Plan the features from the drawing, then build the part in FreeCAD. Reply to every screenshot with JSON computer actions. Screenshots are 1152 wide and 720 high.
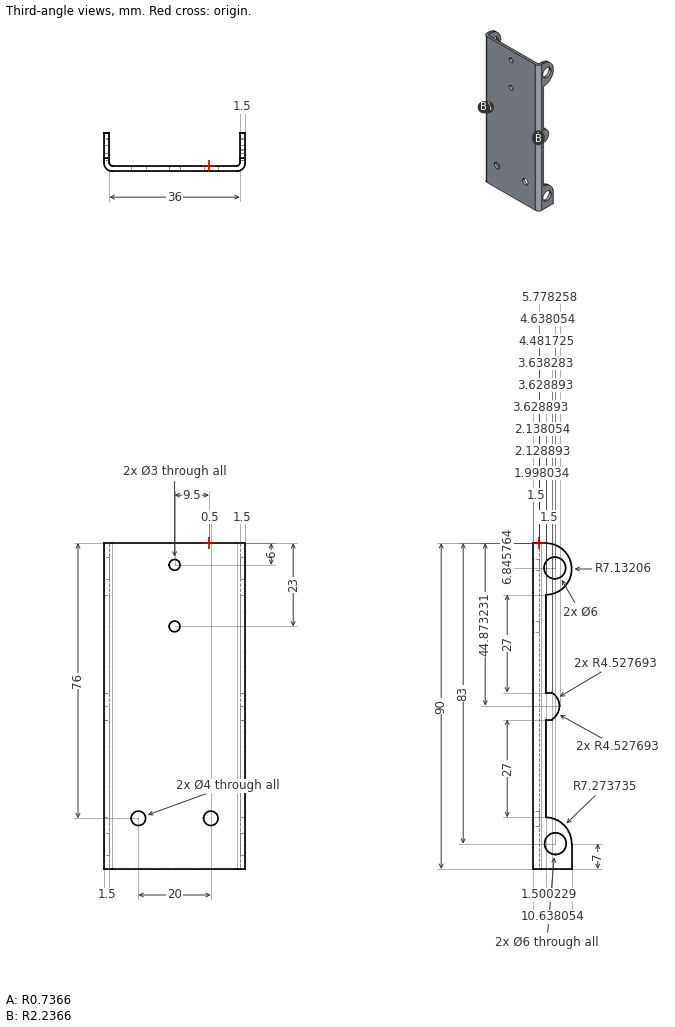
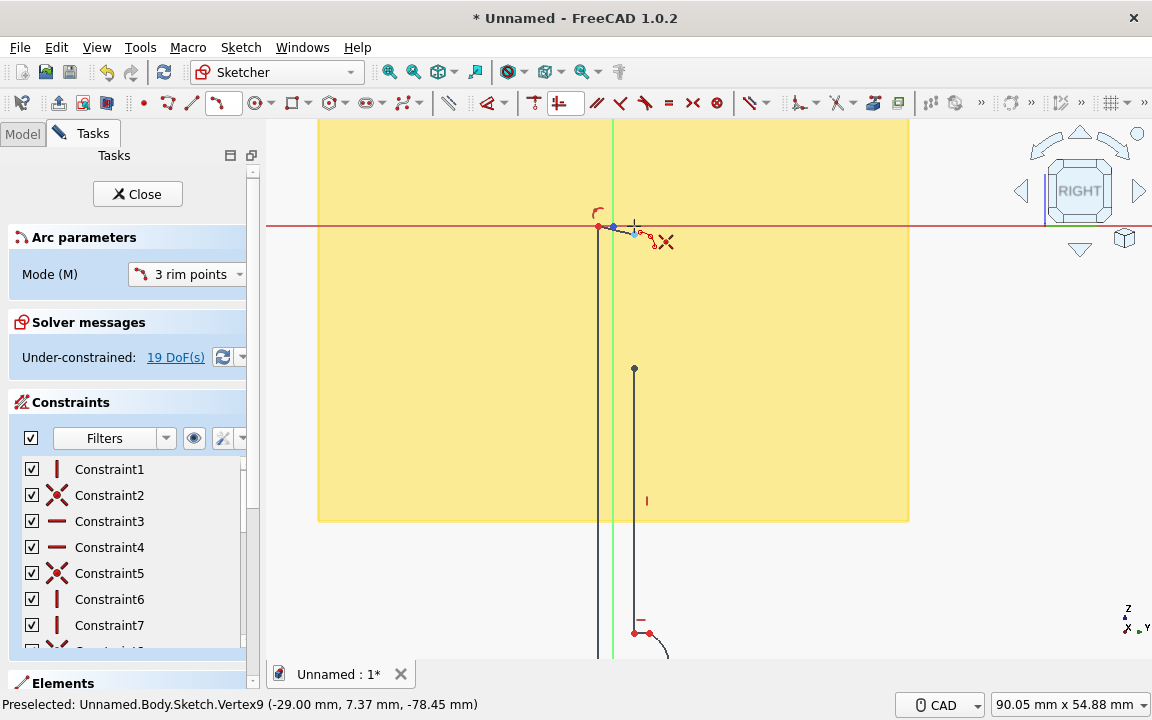
{"action": "left_click", "coordinate": [634, 235]}
{"action": "left_click", "coordinate": [634, 368]}
{"action": "left_click", "coordinate": [703, 296]}
{"action": "key", "text": "Escape"}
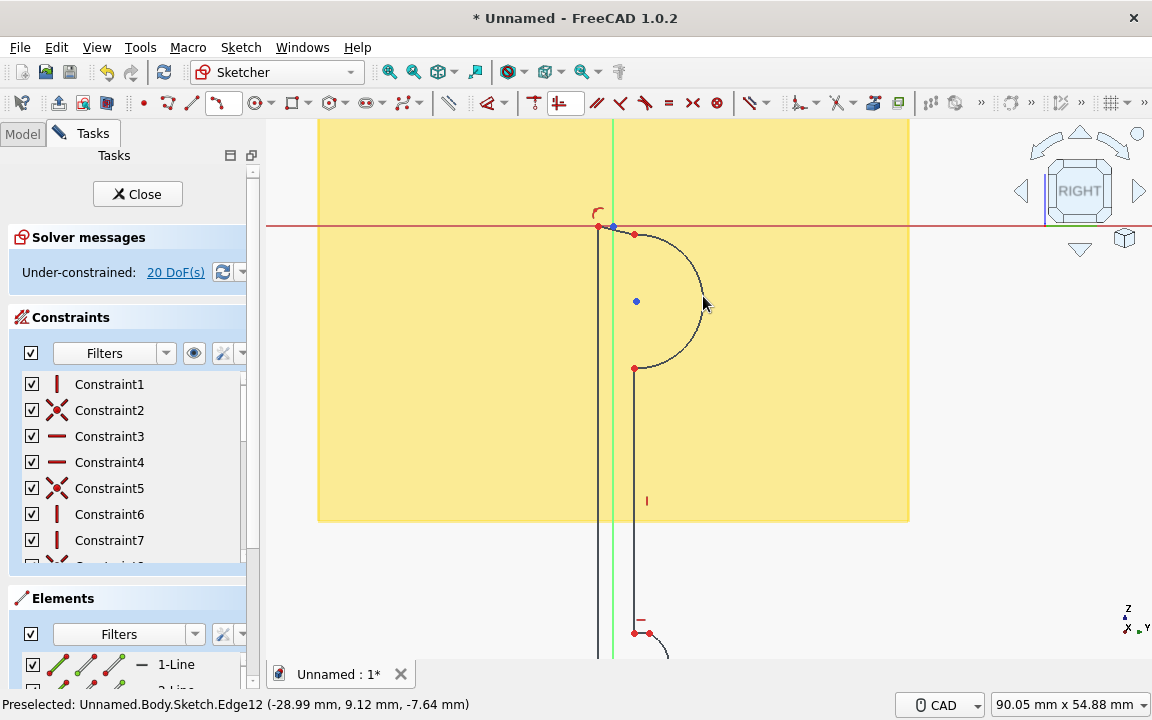
{"action": "scroll", "coordinate": [634, 226], "scroll_direction": "down", "scroll_amount": 5}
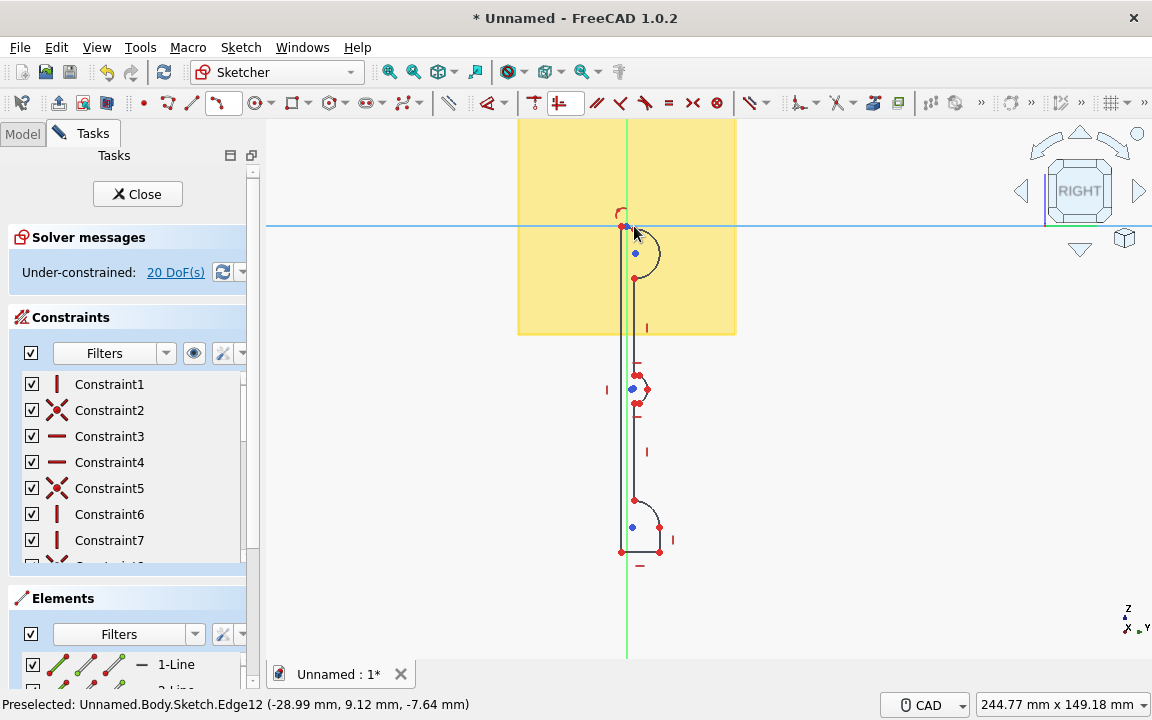
{"action": "scroll", "coordinate": [660, 535], "scroll_direction": "up", "scroll_amount": 4}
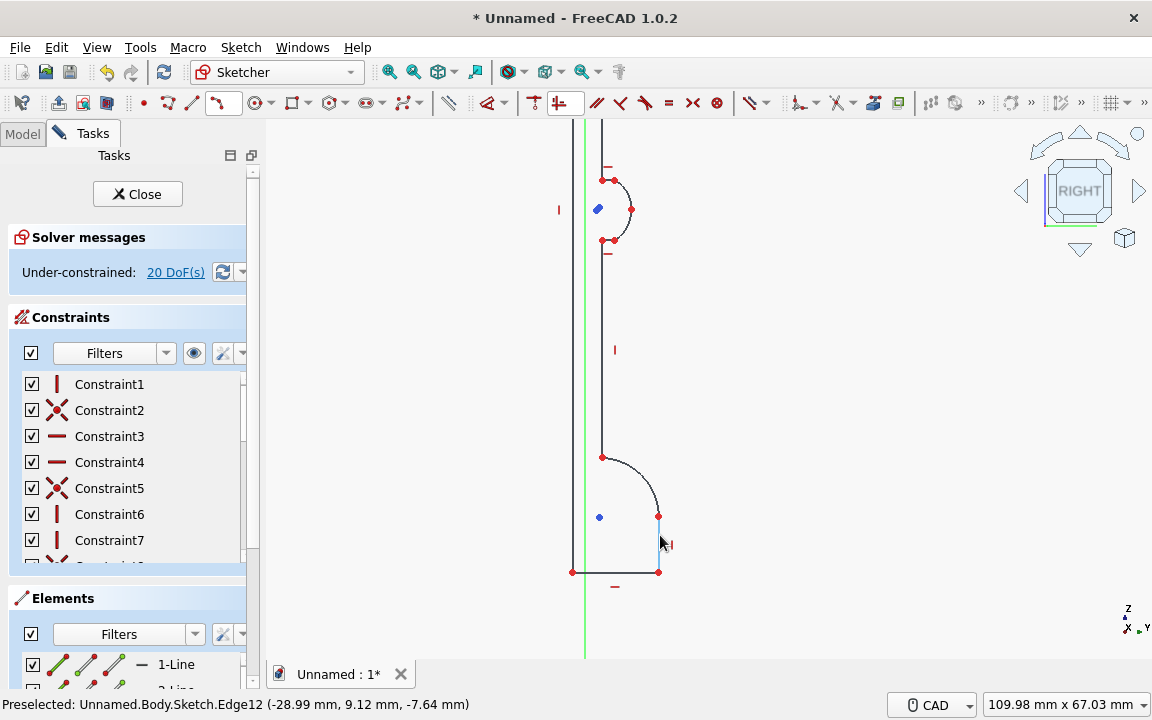
{"action": "left_click", "coordinate": [659, 534]}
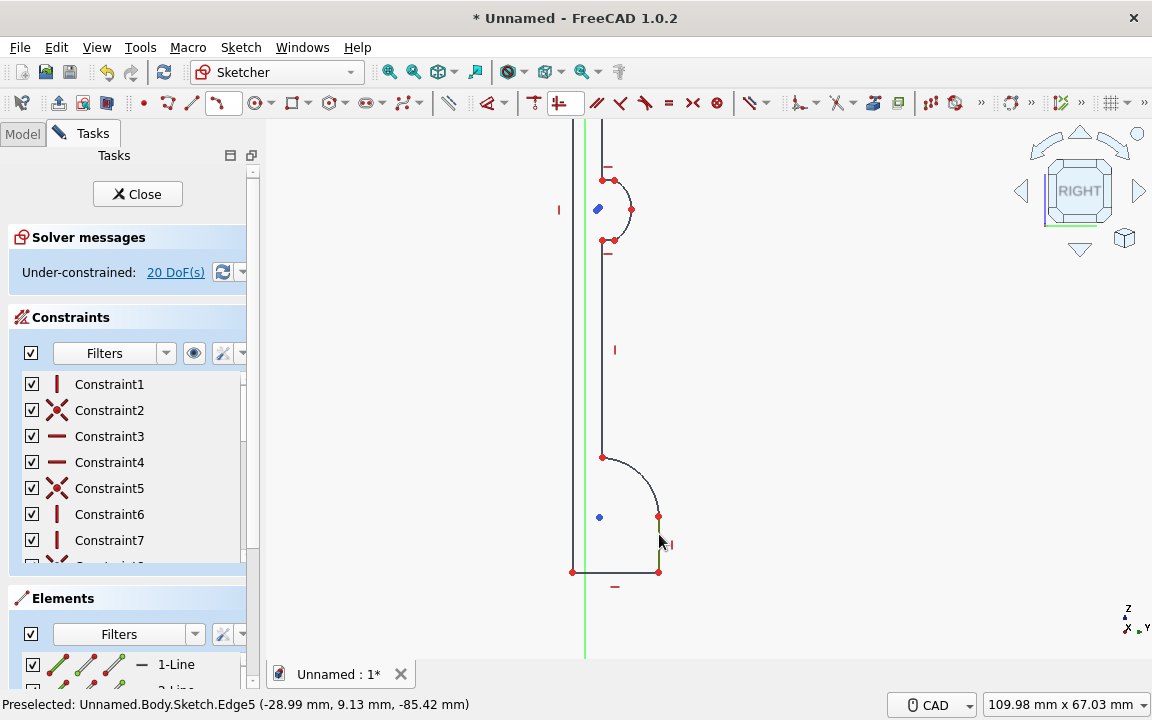
{"action": "left_click", "coordinate": [653, 491]}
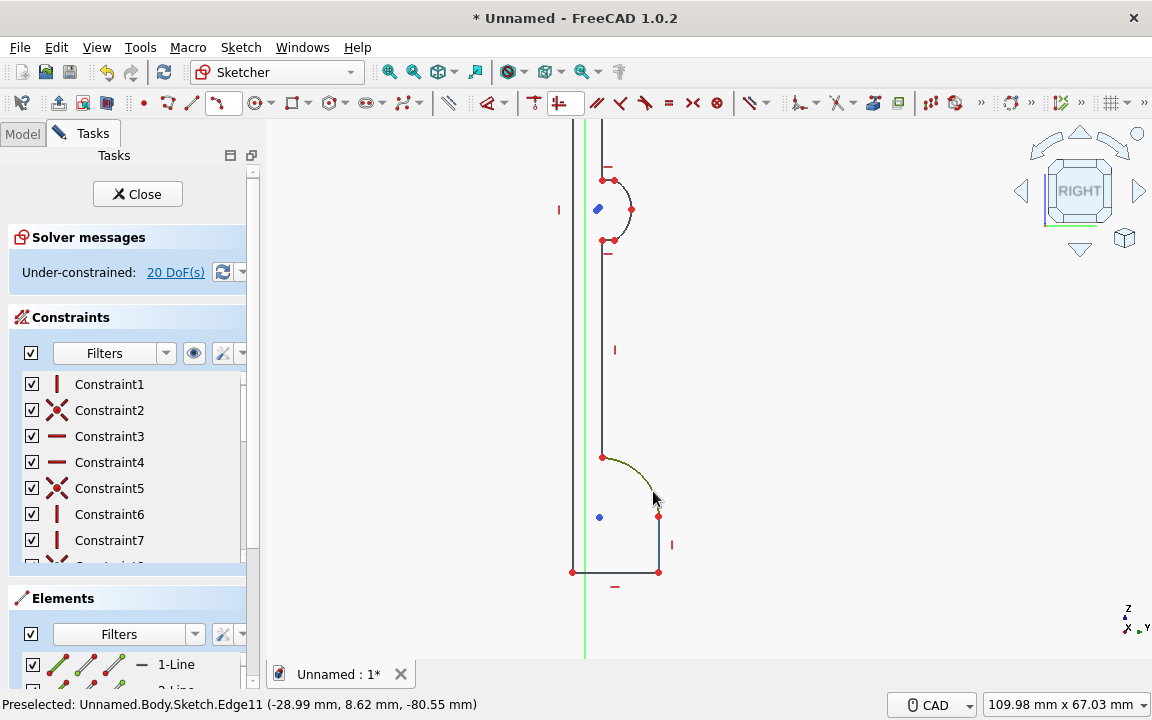
{"action": "key", "text": "t"}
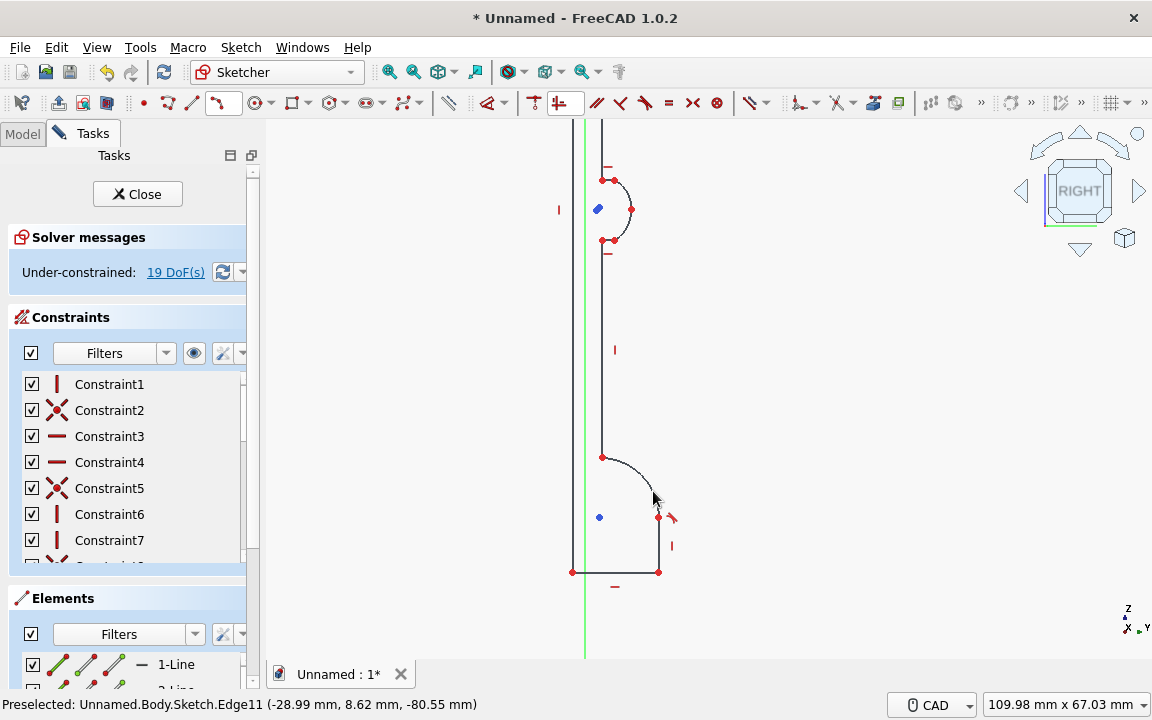
{"action": "scroll", "coordinate": [660, 536], "scroll_direction": "down", "scroll_amount": 4}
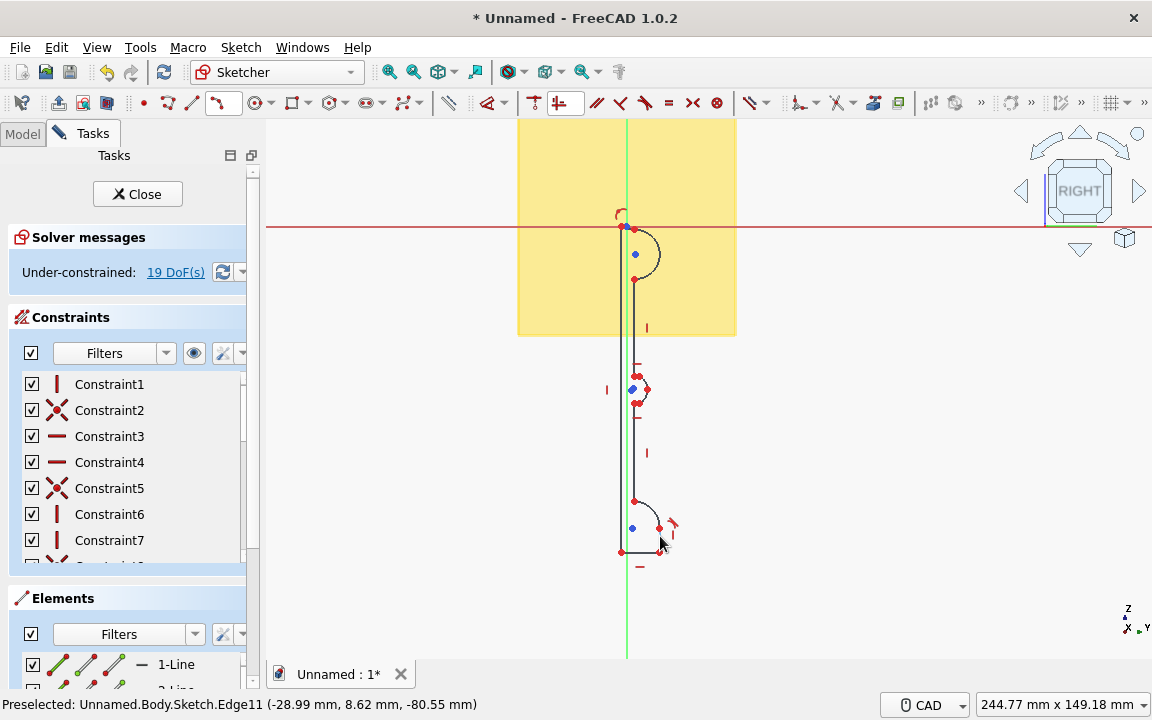
{"action": "scroll", "coordinate": [626, 228], "scroll_direction": "up", "scroll_amount": 5}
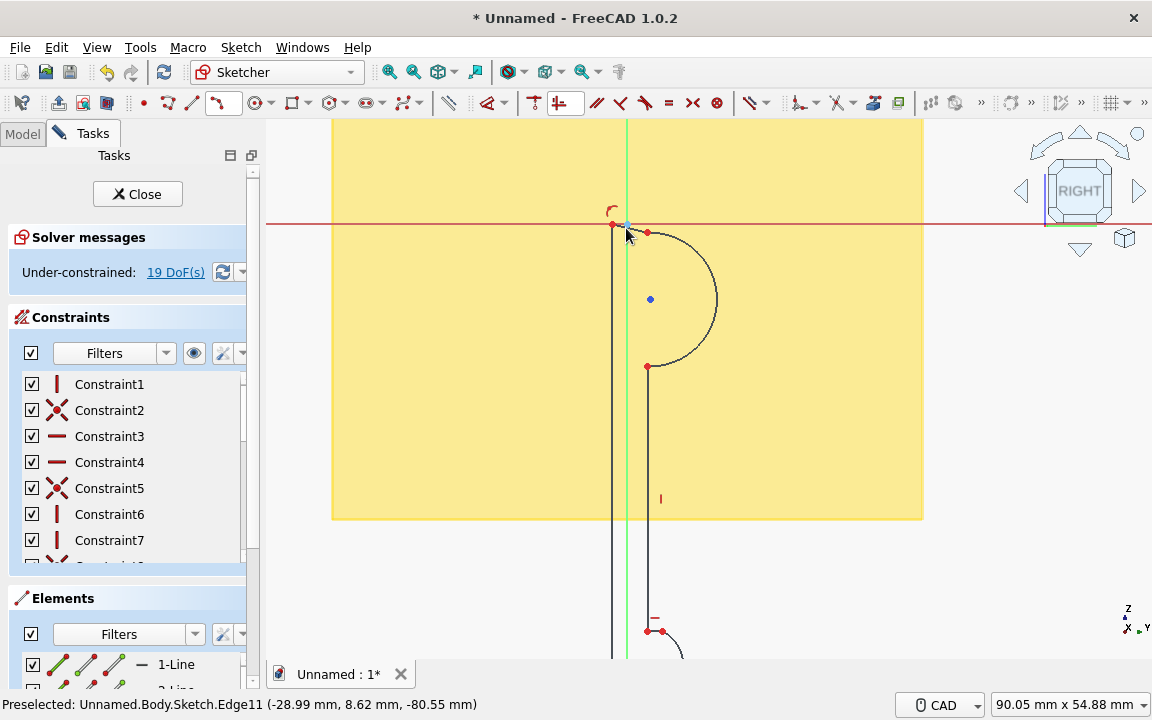
{"action": "left_click", "coordinate": [630, 229]}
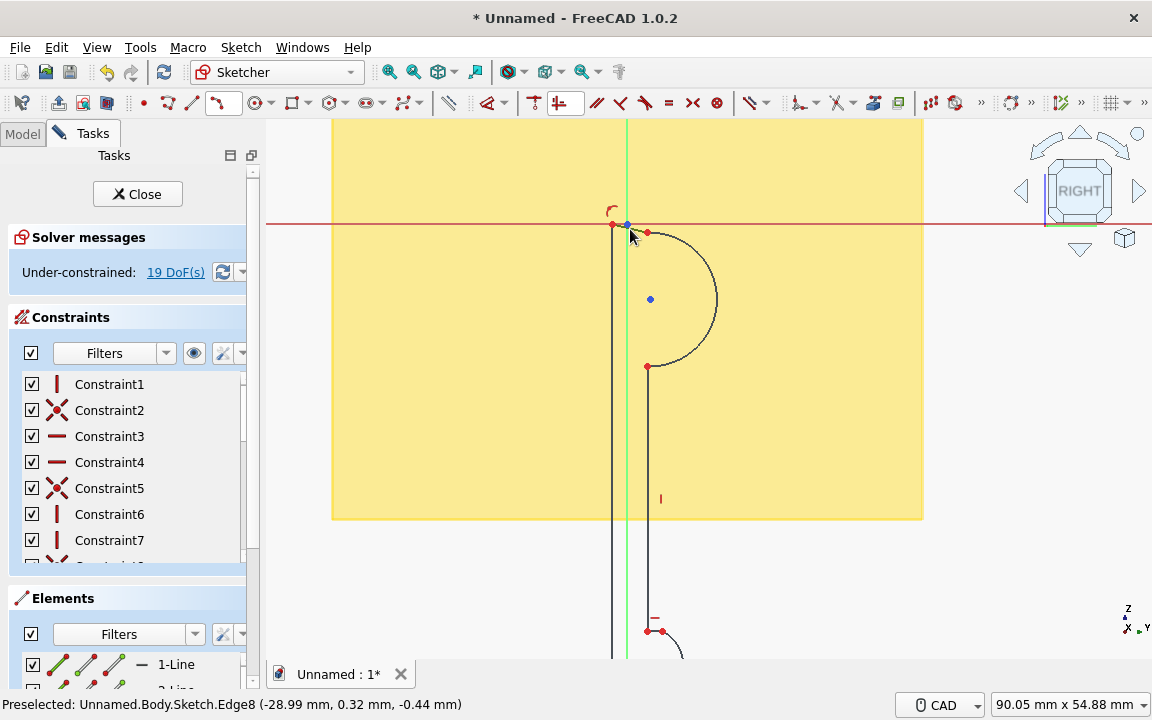
{"action": "key", "text": "h"}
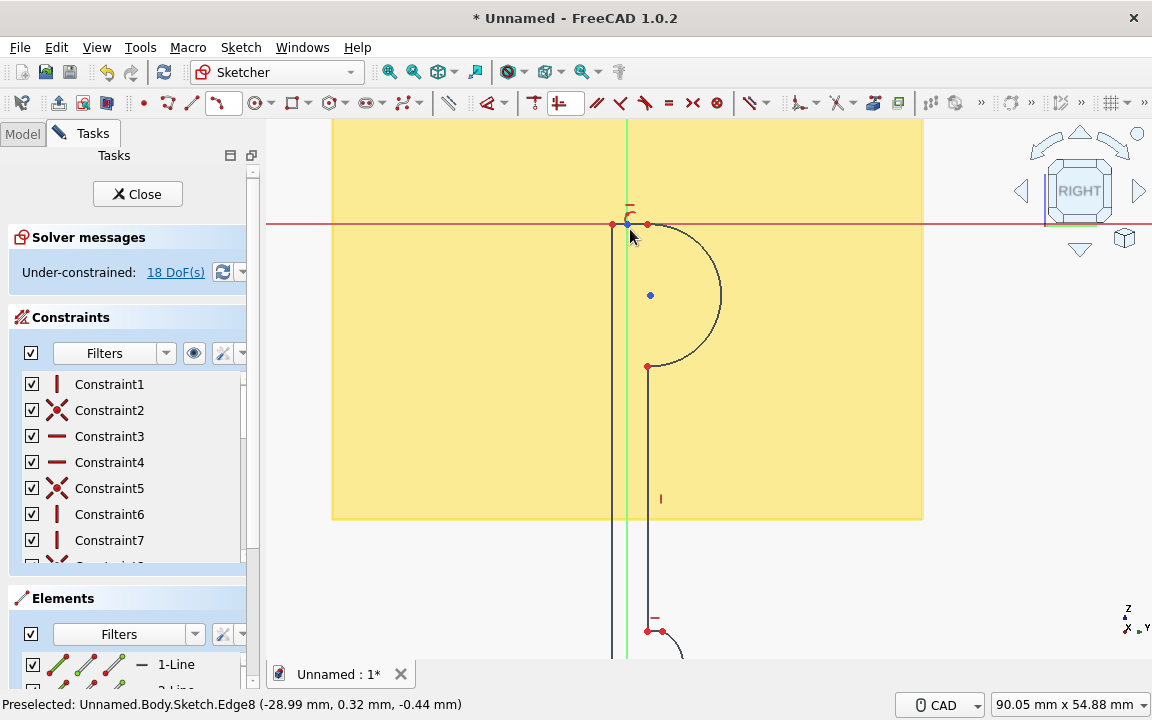
{"action": "scroll", "coordinate": [626, 227], "scroll_direction": "down", "scroll_amount": 5}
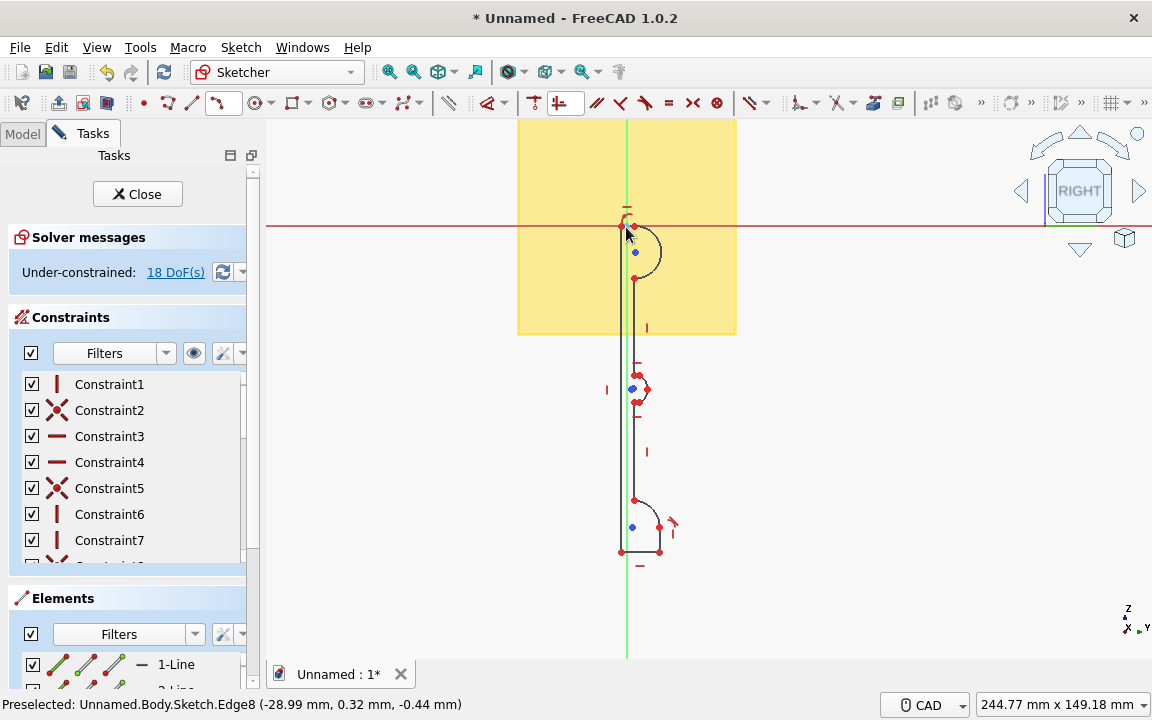
{"action": "scroll", "coordinate": [647, 384], "scroll_direction": "up", "scroll_amount": 6}